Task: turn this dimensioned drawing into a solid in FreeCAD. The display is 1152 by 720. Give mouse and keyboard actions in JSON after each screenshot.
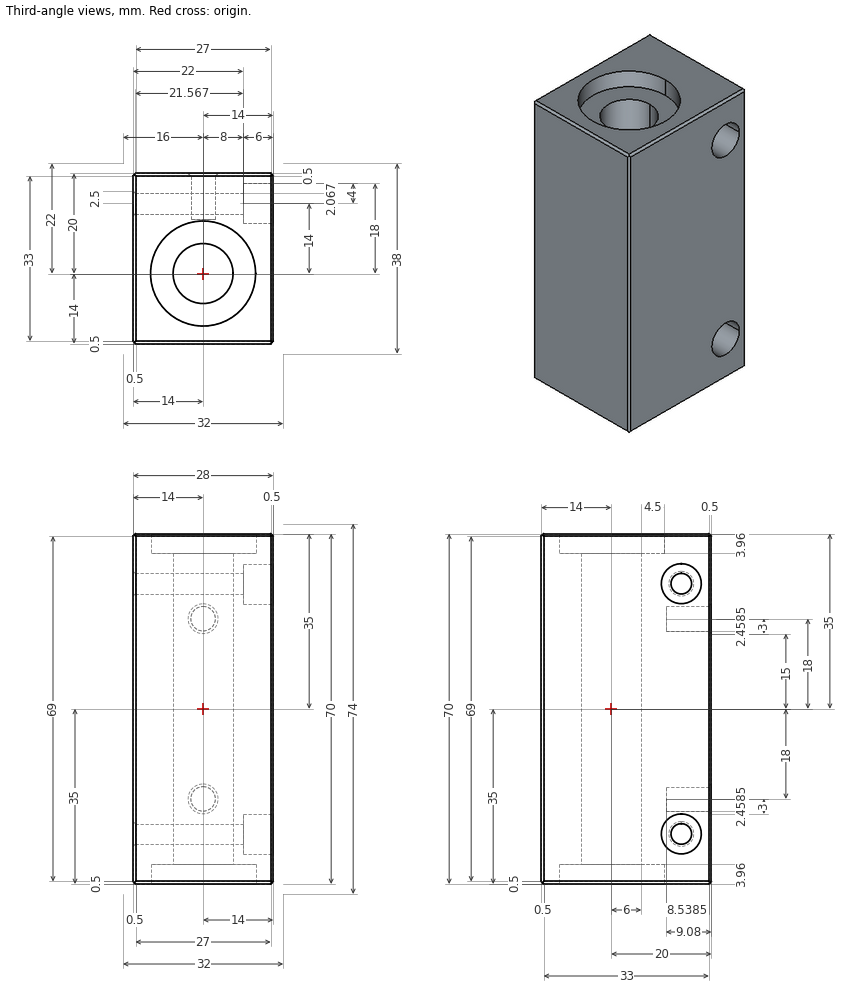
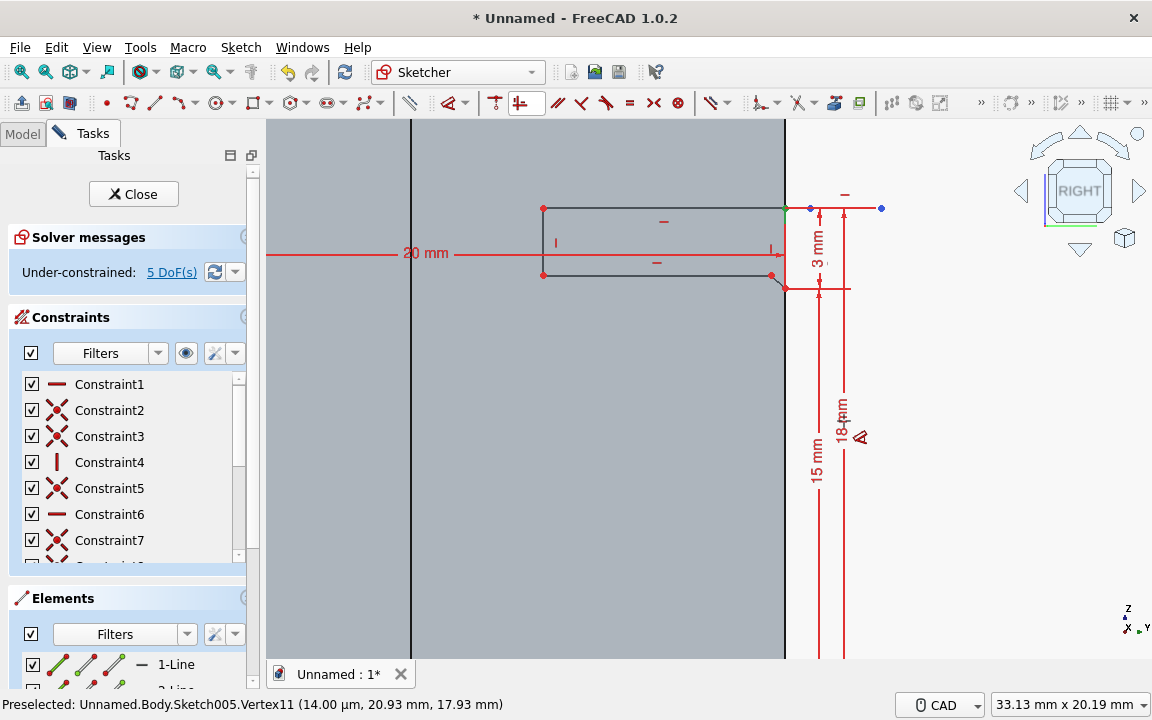
{"action": "left_click", "coordinate": [713, 208]}
{"action": "left_click", "coordinate": [664, 174]}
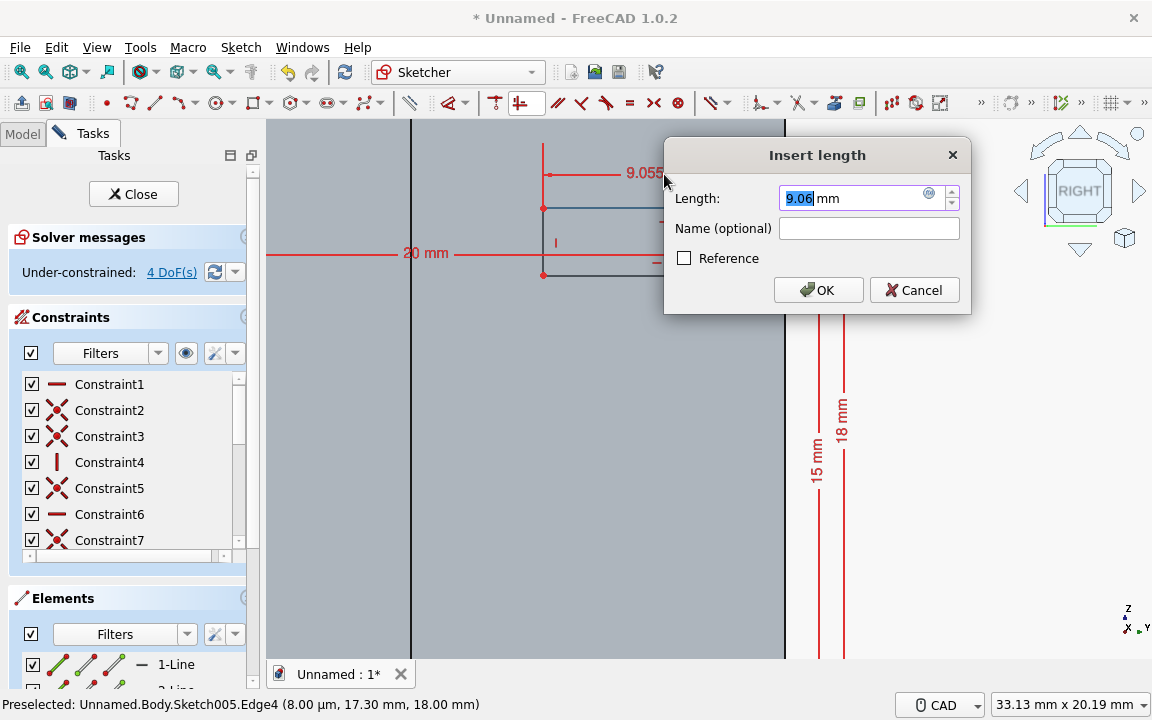
{"action": "type", "text": "9.08"}
{"action": "key", "text": "Return"}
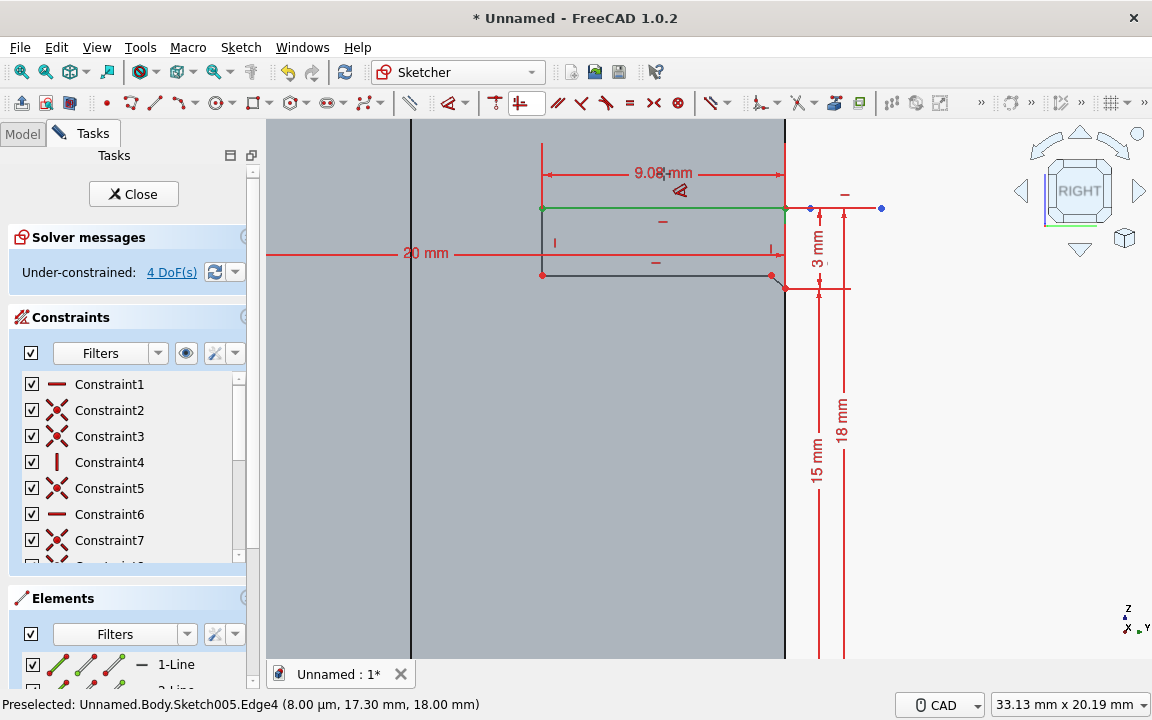
{"action": "left_click", "coordinate": [611, 276]}
{"action": "left_click", "coordinate": [657, 242]}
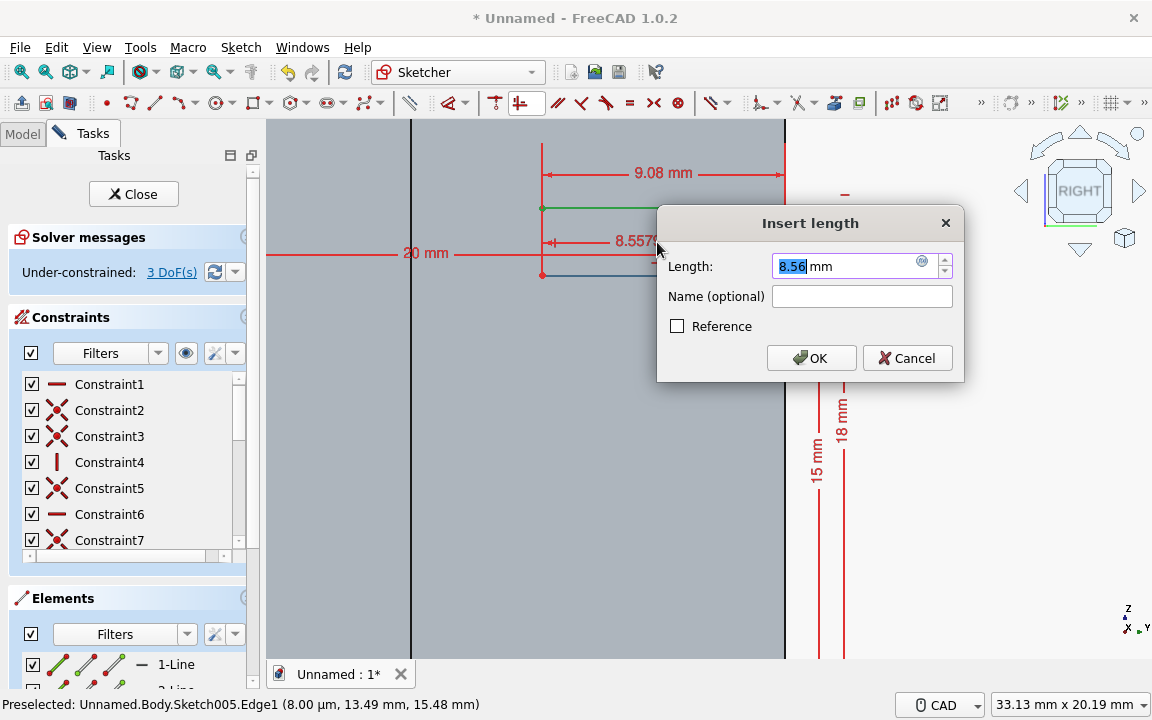
{"action": "type", "text": "8.5385"}
{"action": "key", "text": "Return"}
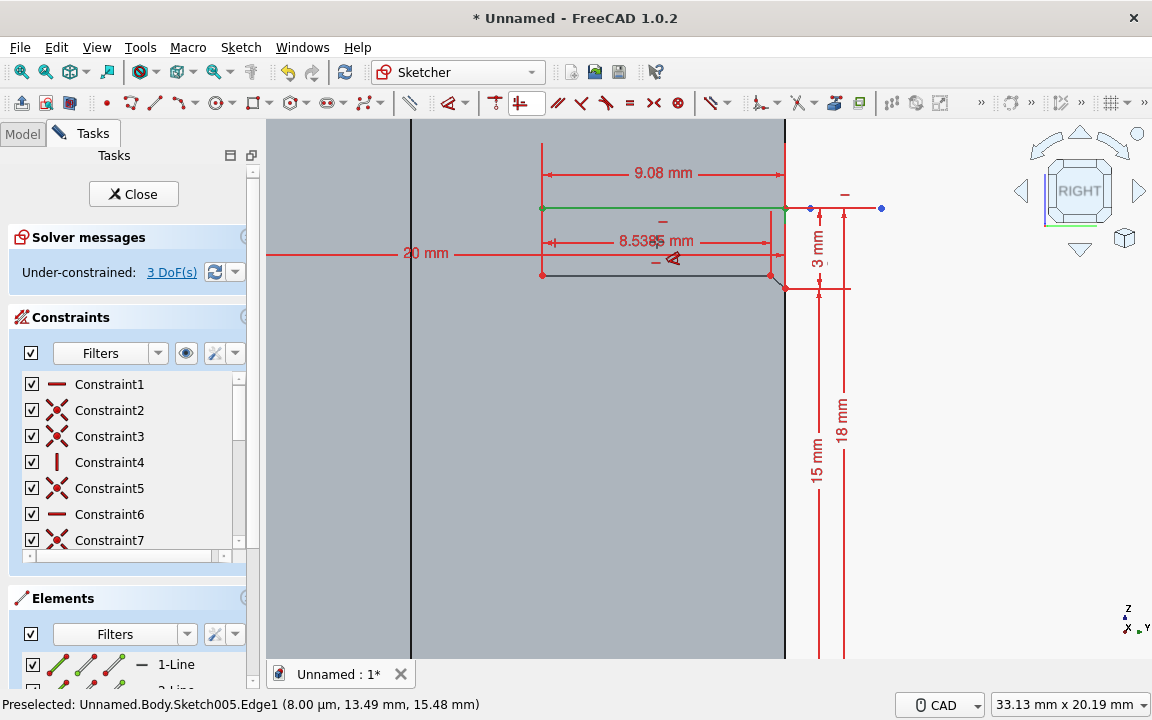
{"action": "left_click", "coordinate": [542, 229]}
{"action": "left_click", "coordinate": [508, 242]}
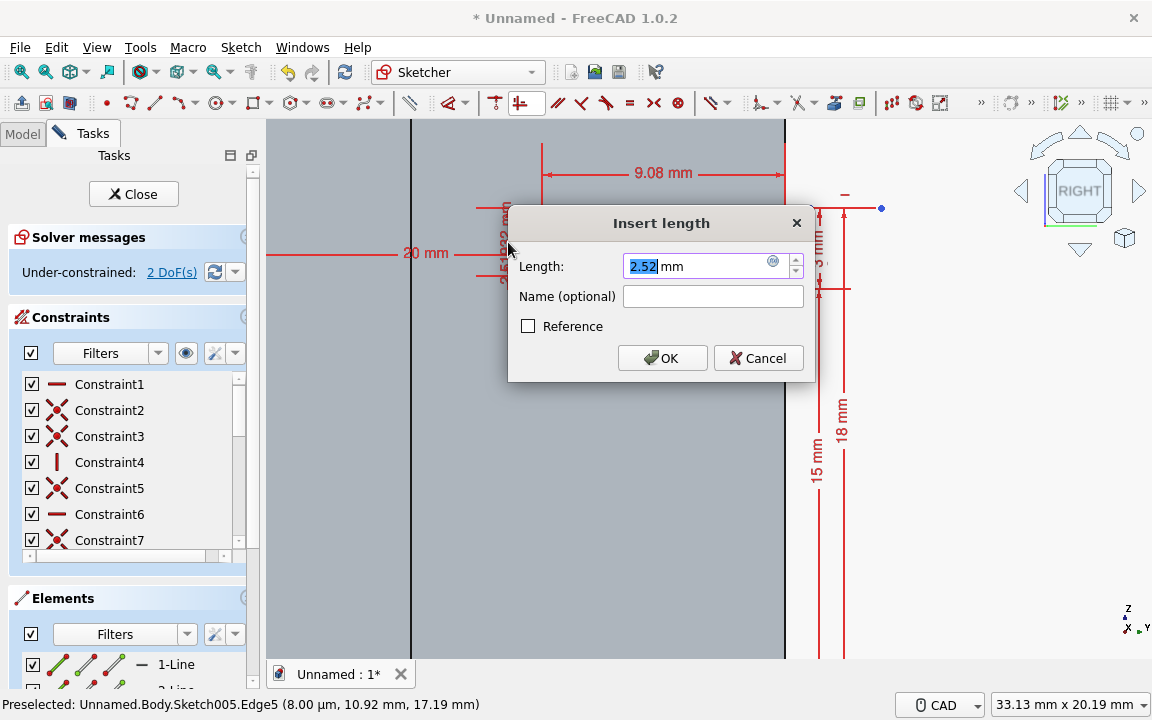
{"action": "type", "text": "2.4585"}
{"action": "key", "text": "Return"}
{"action": "key", "text": "Escape"}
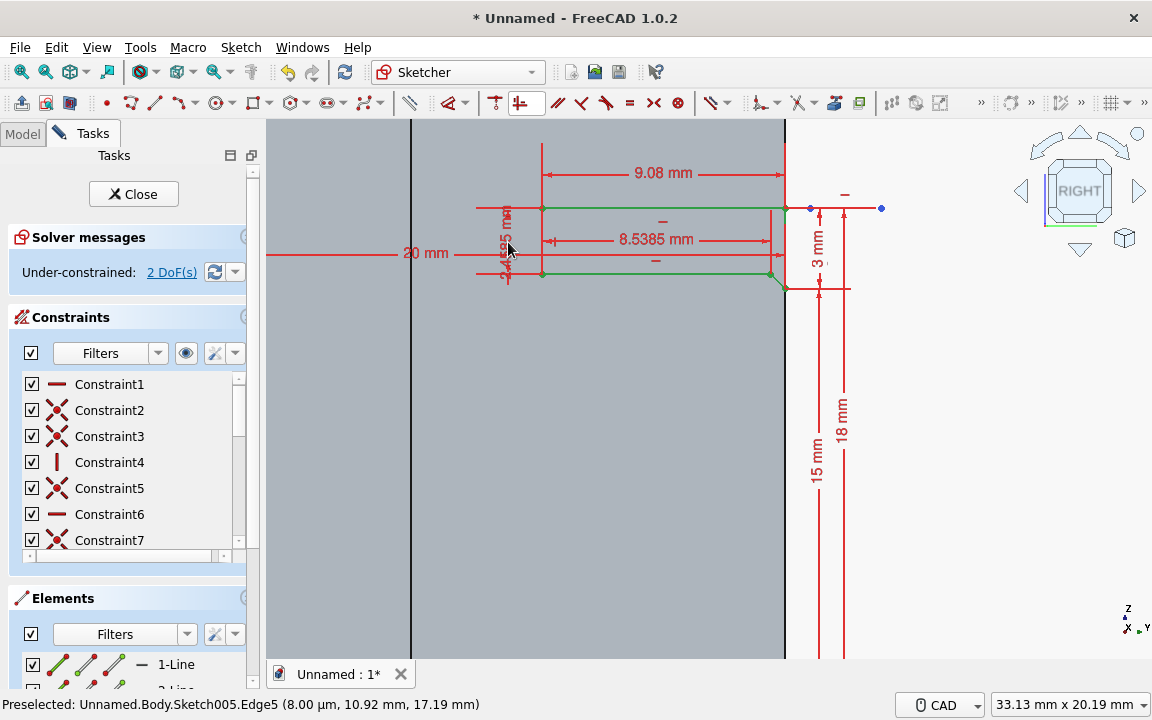
{"action": "left_click", "coordinate": [134, 194]}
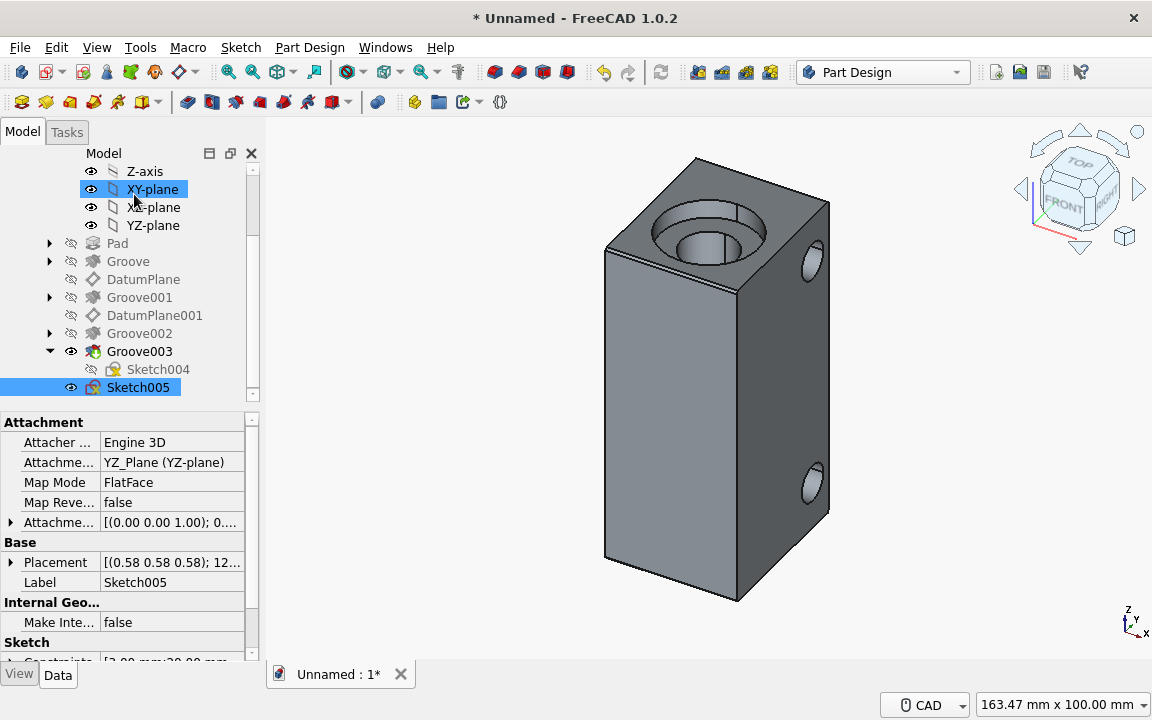
{"action": "left_click", "coordinate": [236, 102]}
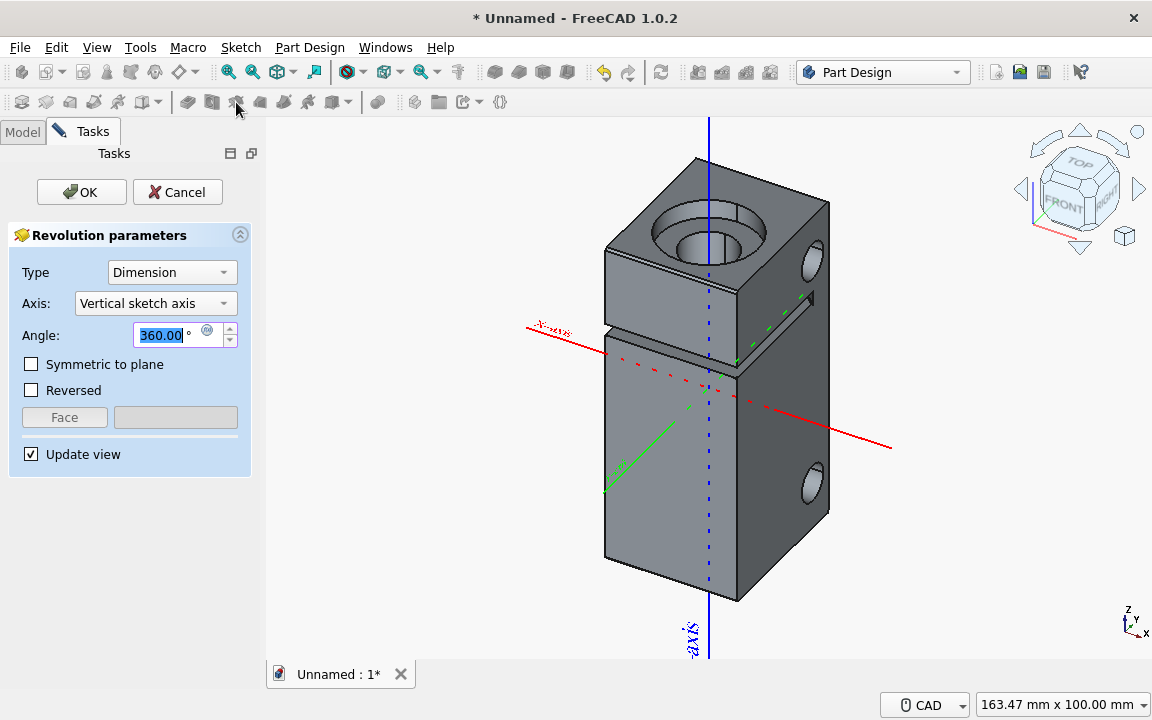
{"action": "left_click", "coordinate": [156, 304]}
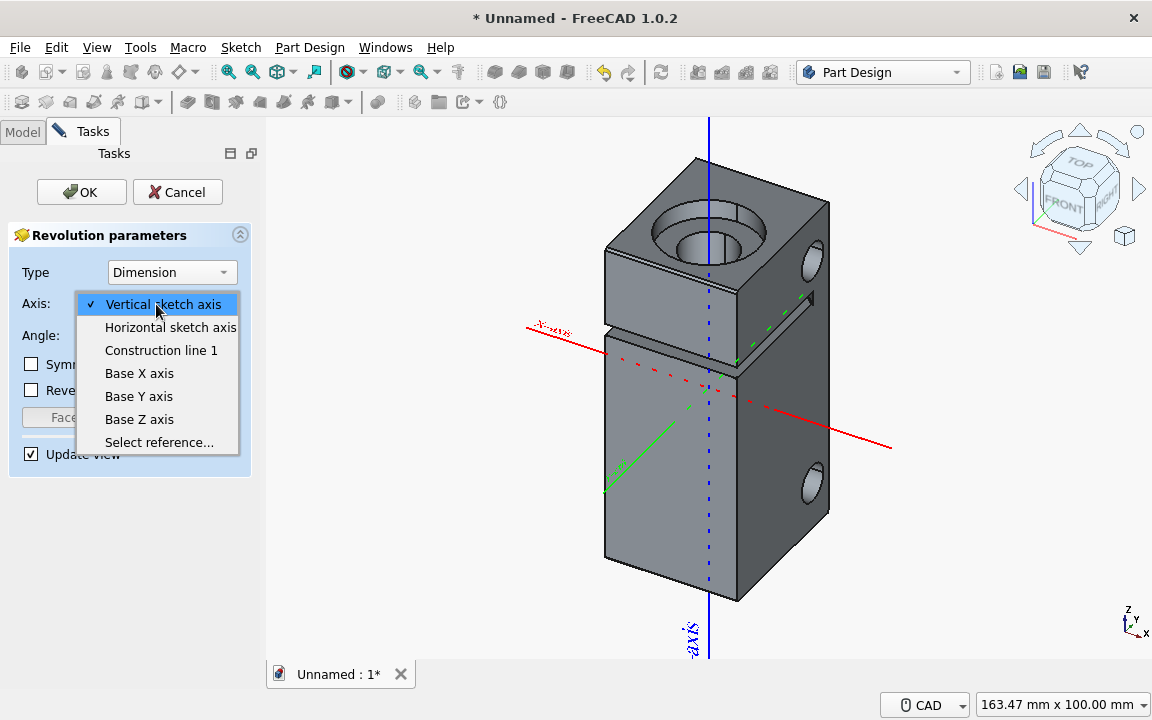
{"action": "left_click", "coordinate": [156, 350]}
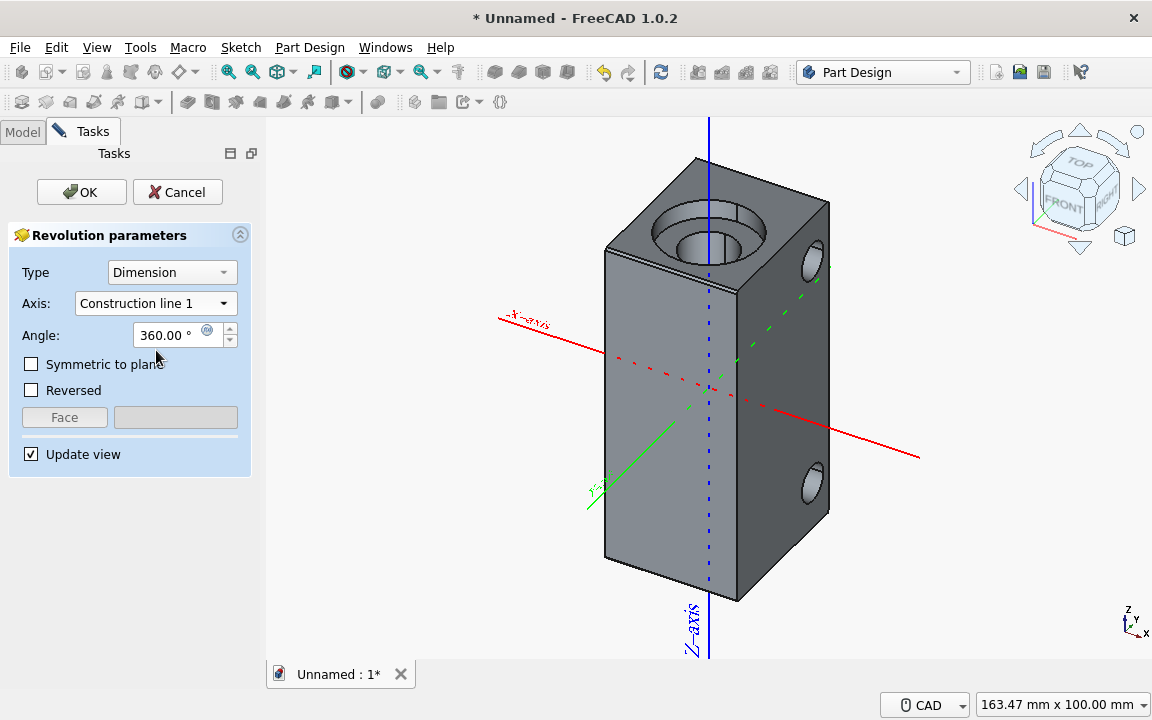
{"action": "left_click", "coordinate": [82, 192]}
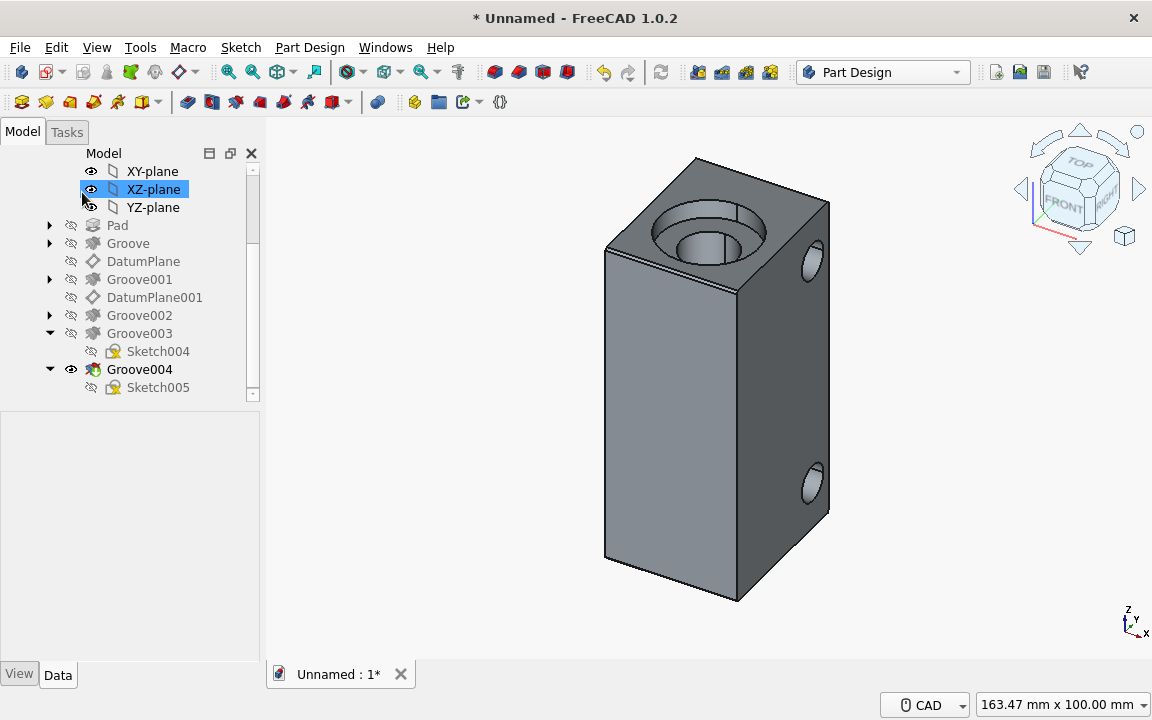
{"action": "scroll", "coordinate": [160, 275], "scroll_direction": "down", "scroll_amount": 3}